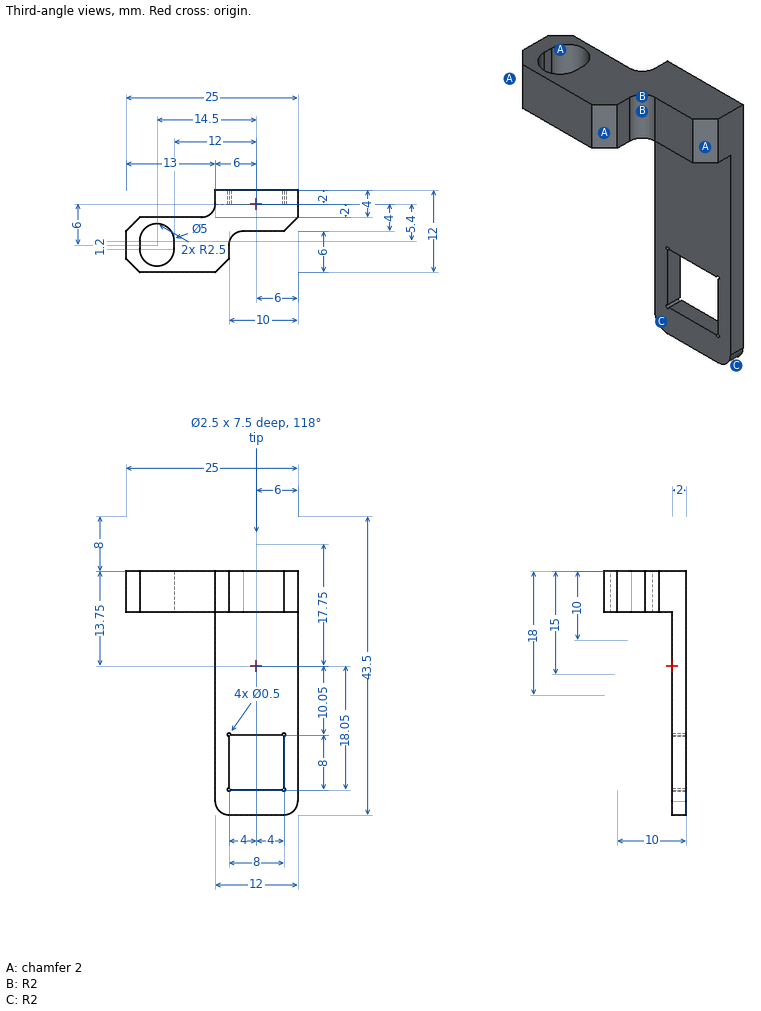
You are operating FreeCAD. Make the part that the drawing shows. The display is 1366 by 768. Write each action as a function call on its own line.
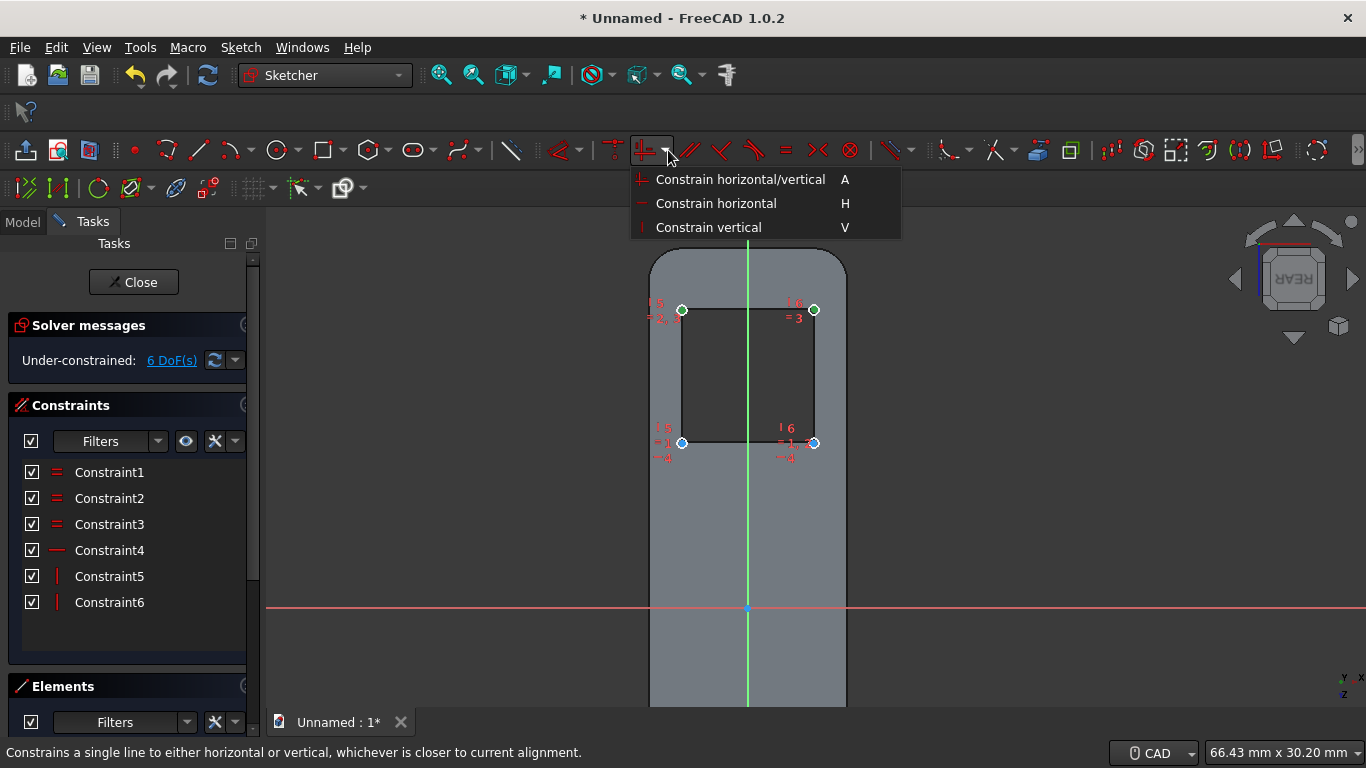
click(766, 203)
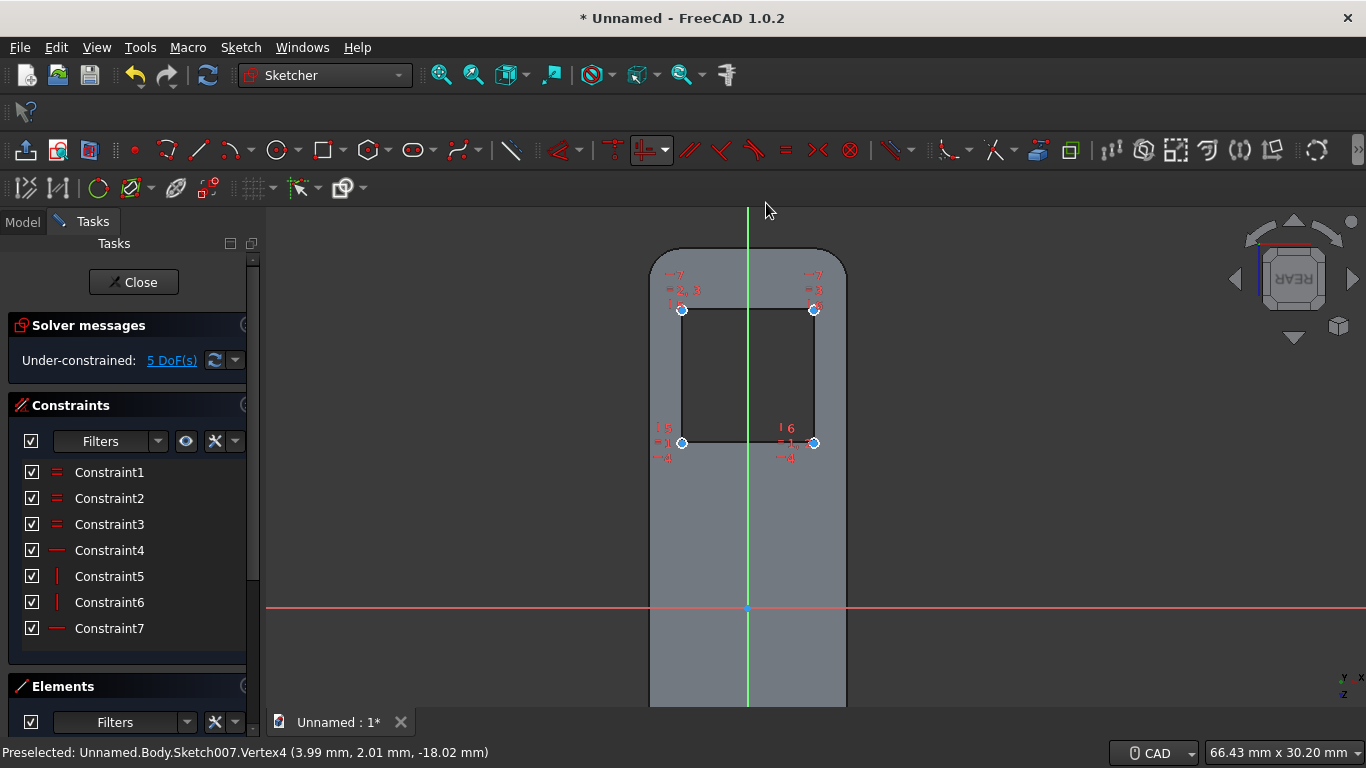
click(558, 150)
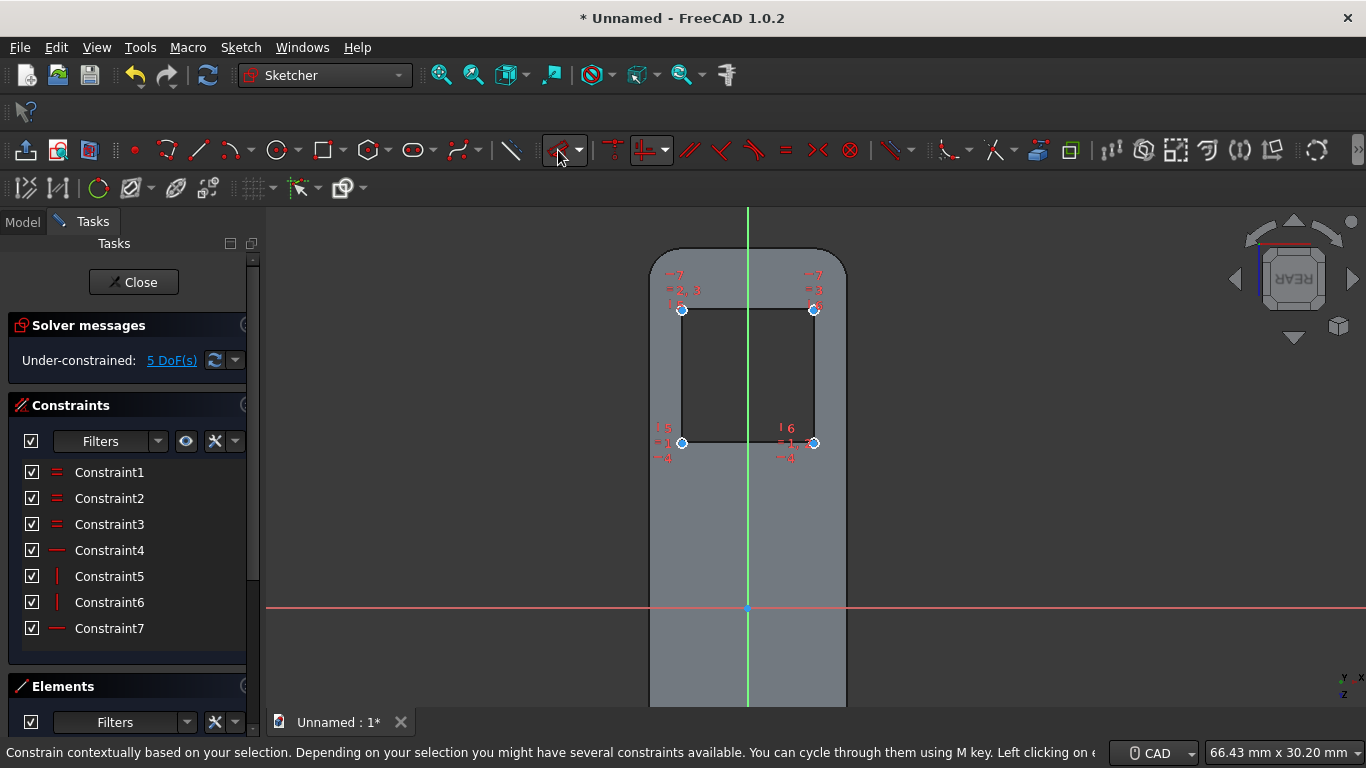
scroll(677, 443, up, 8)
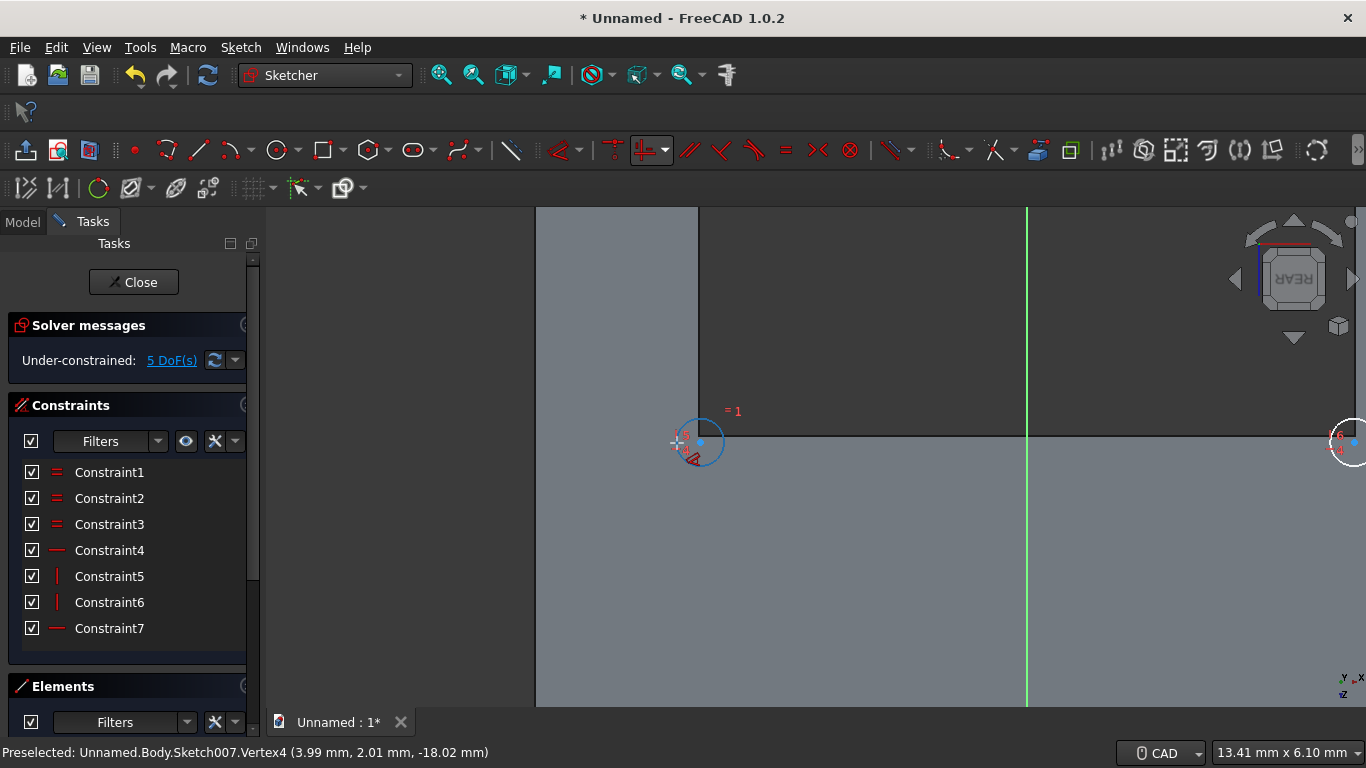
click(677, 442)
click(645, 442)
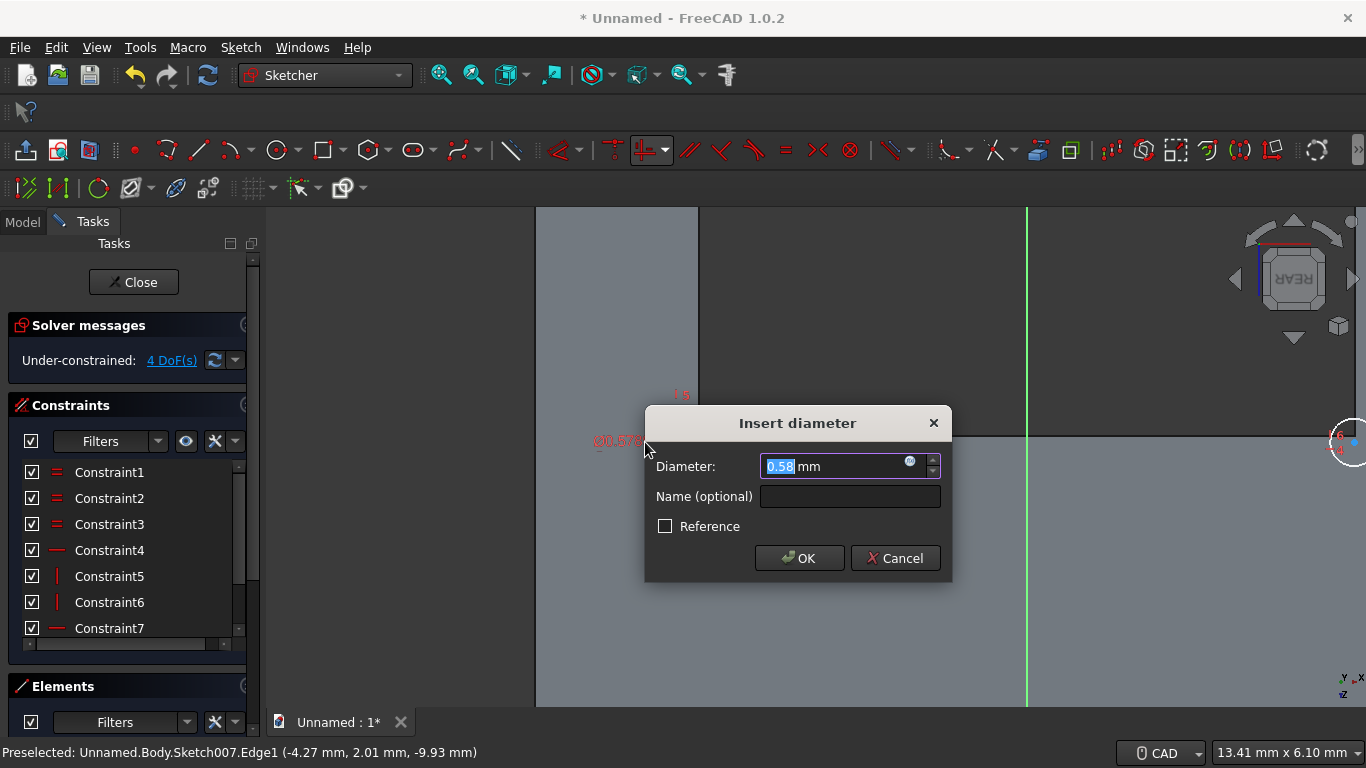
text(0.5)
key(Return)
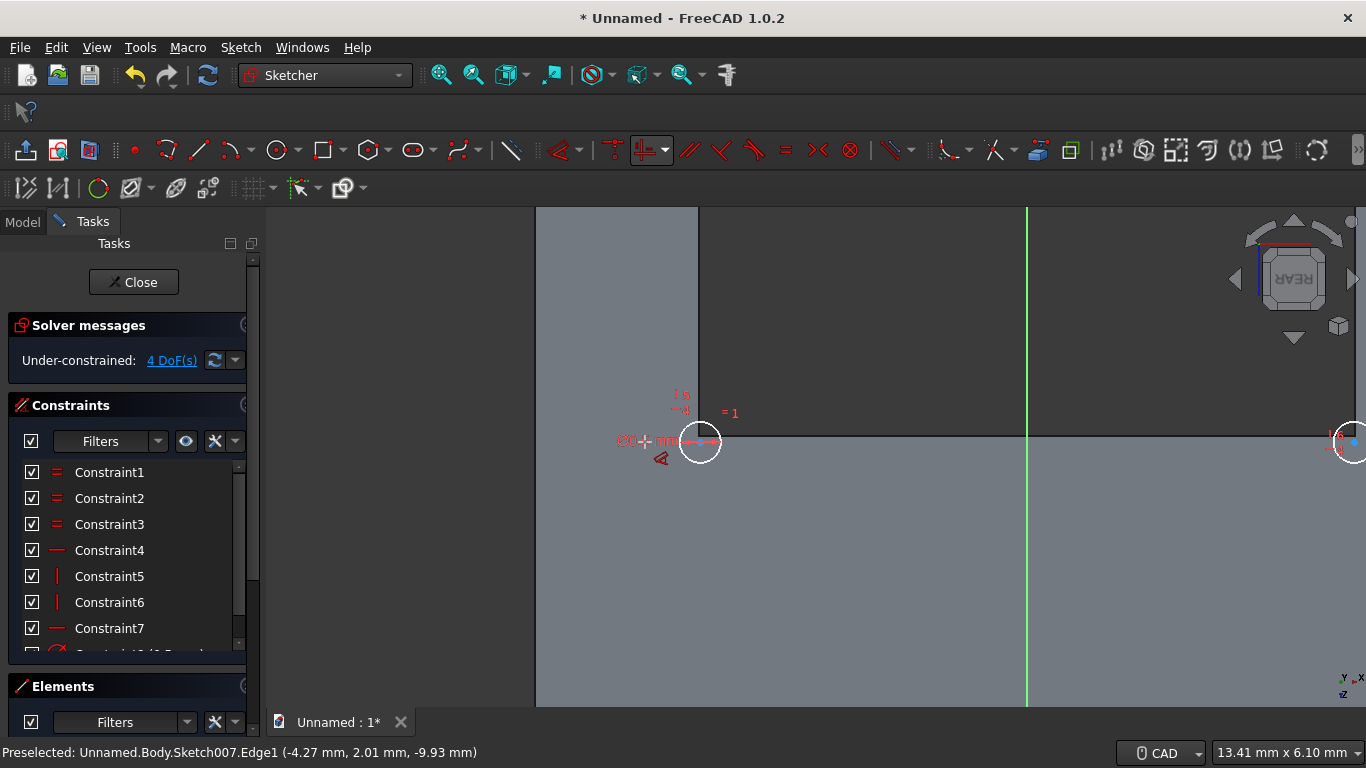
scroll(677, 444, down, 8)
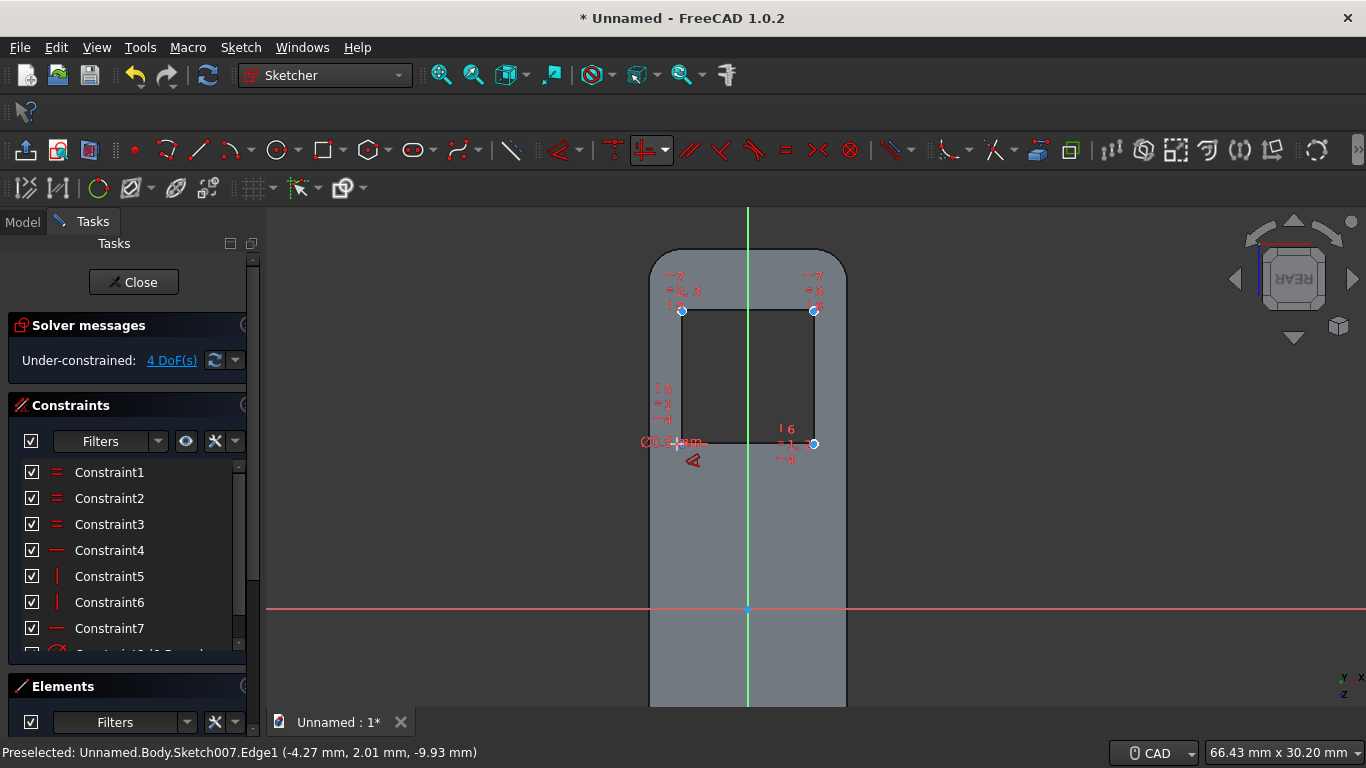
click(682, 444)
click(715, 643)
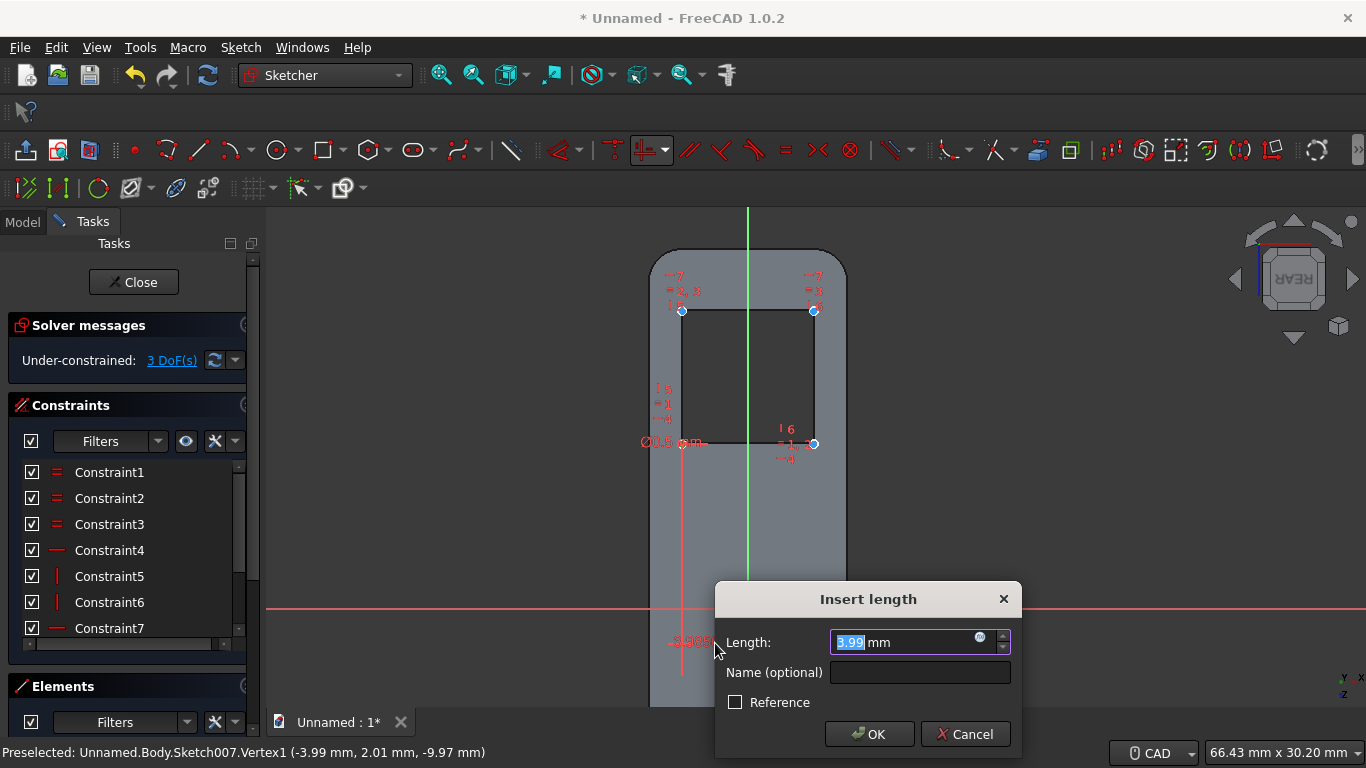
text(4)
key(Return)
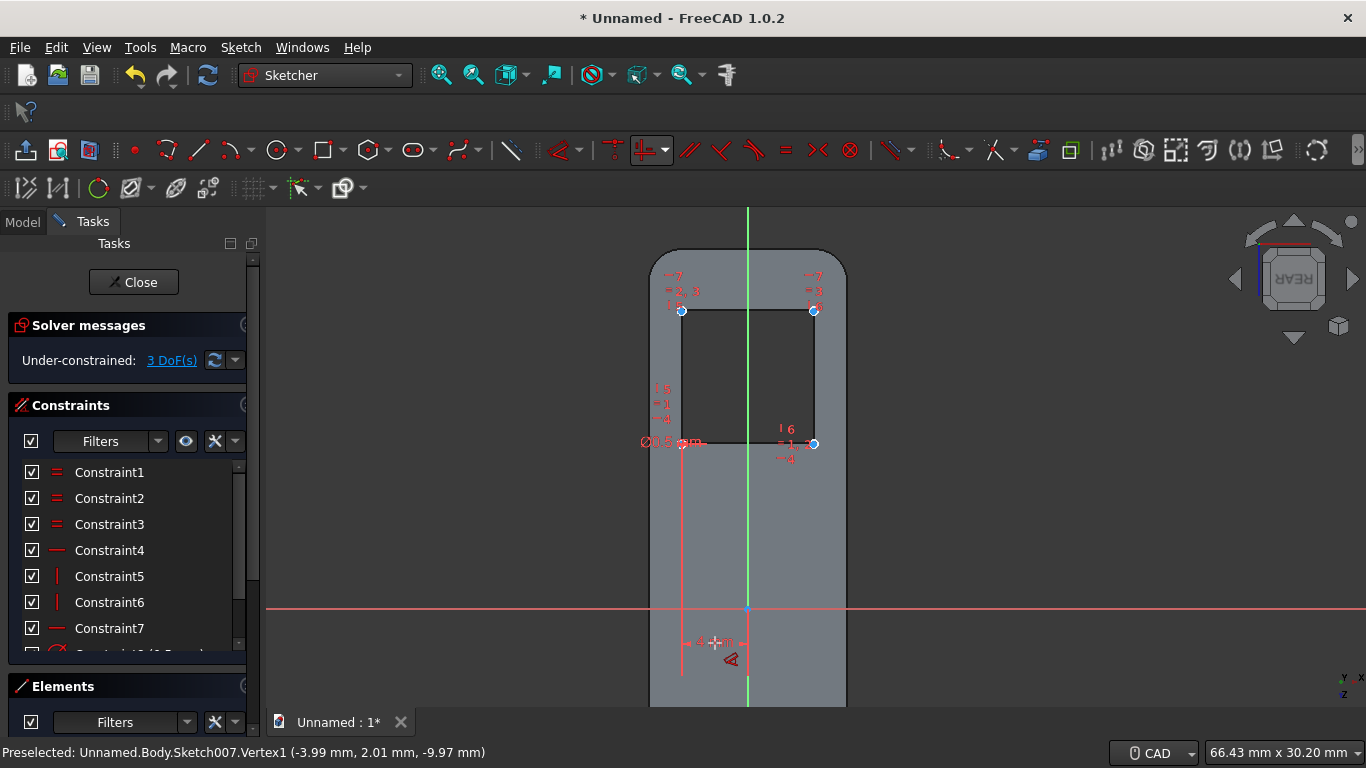
click(814, 444)
click(796, 643)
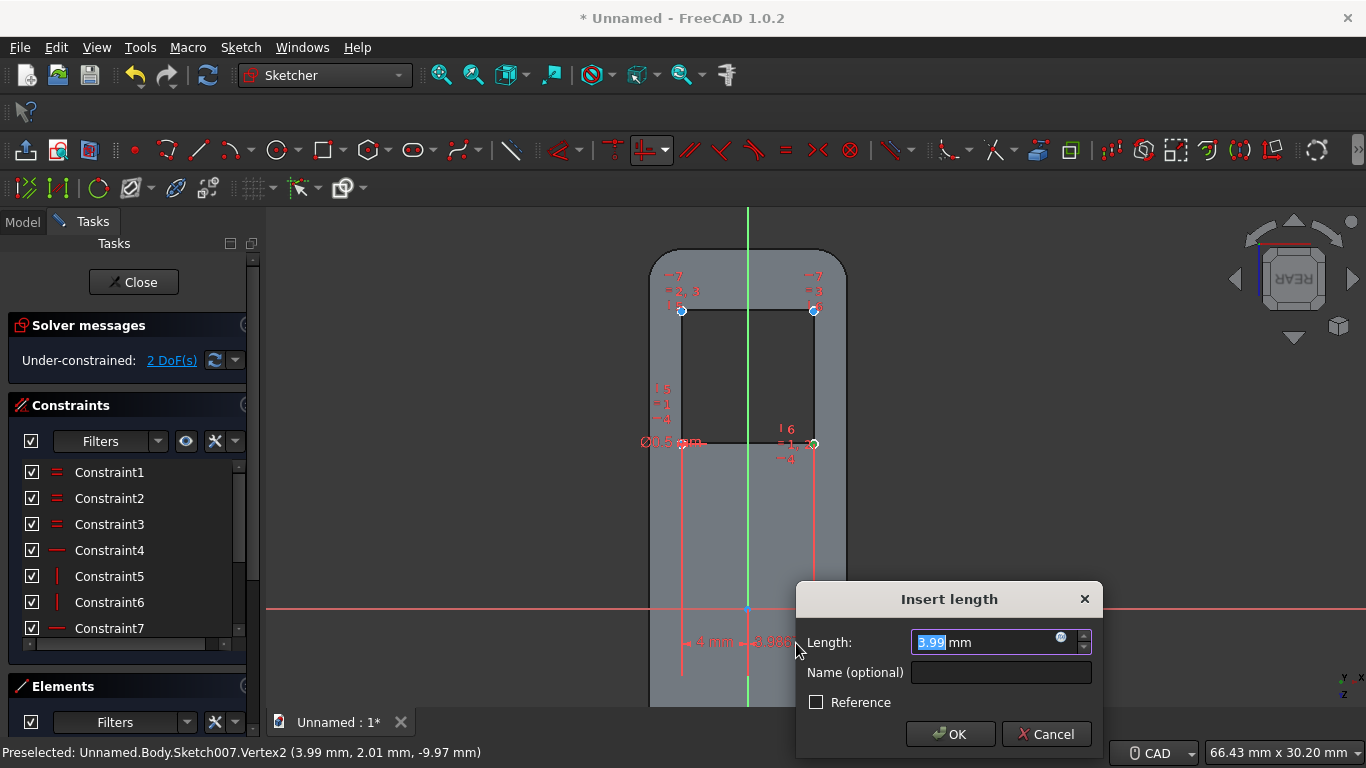
text(4)
key(Return)